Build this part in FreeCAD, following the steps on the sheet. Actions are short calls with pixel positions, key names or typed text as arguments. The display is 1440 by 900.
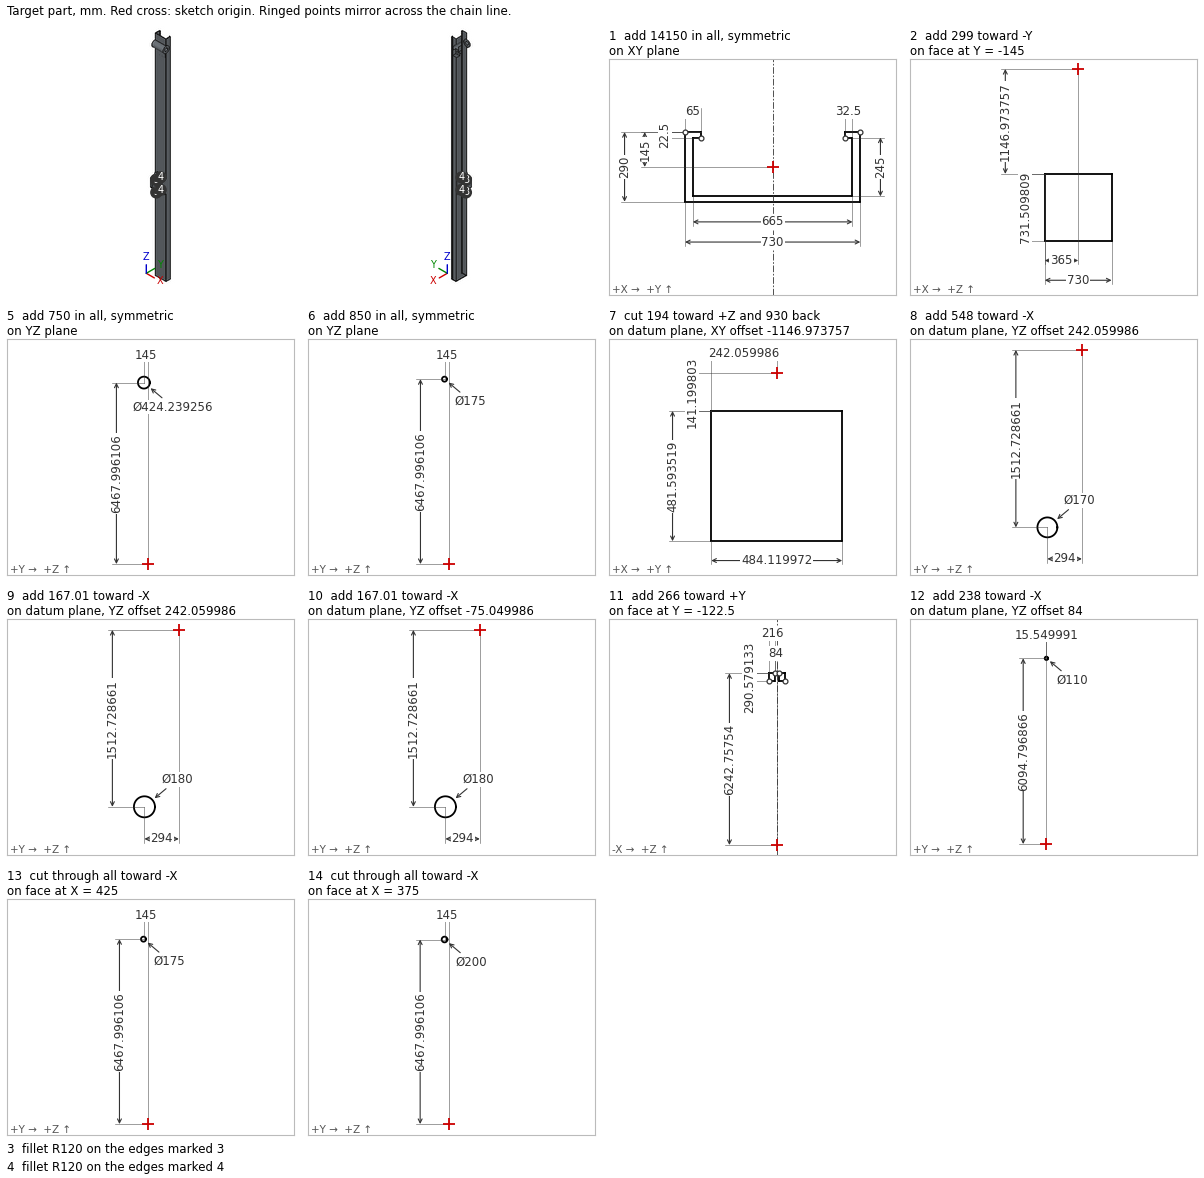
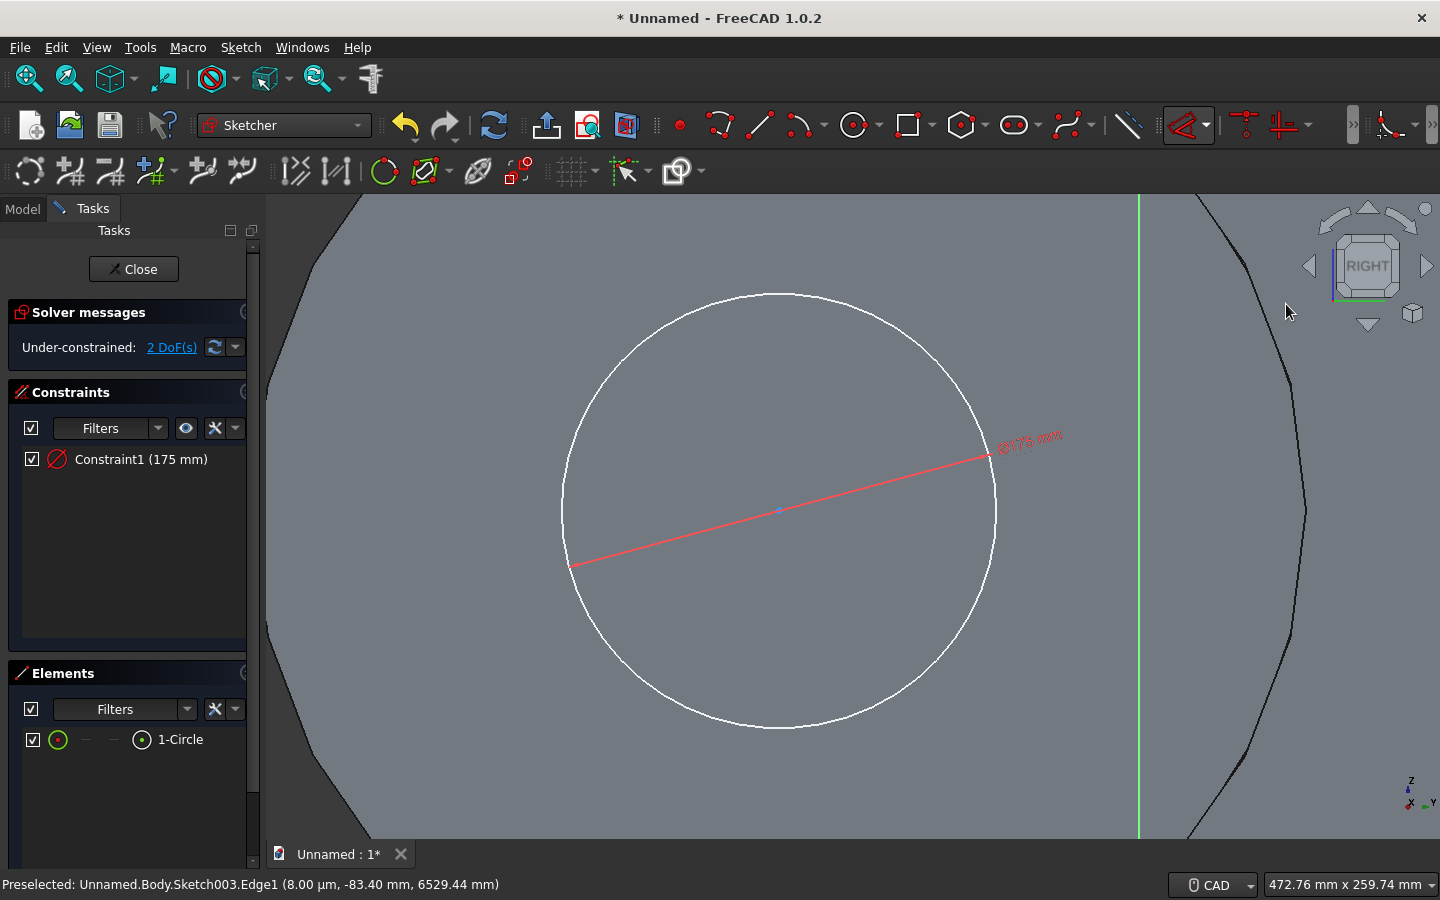
click(779, 511)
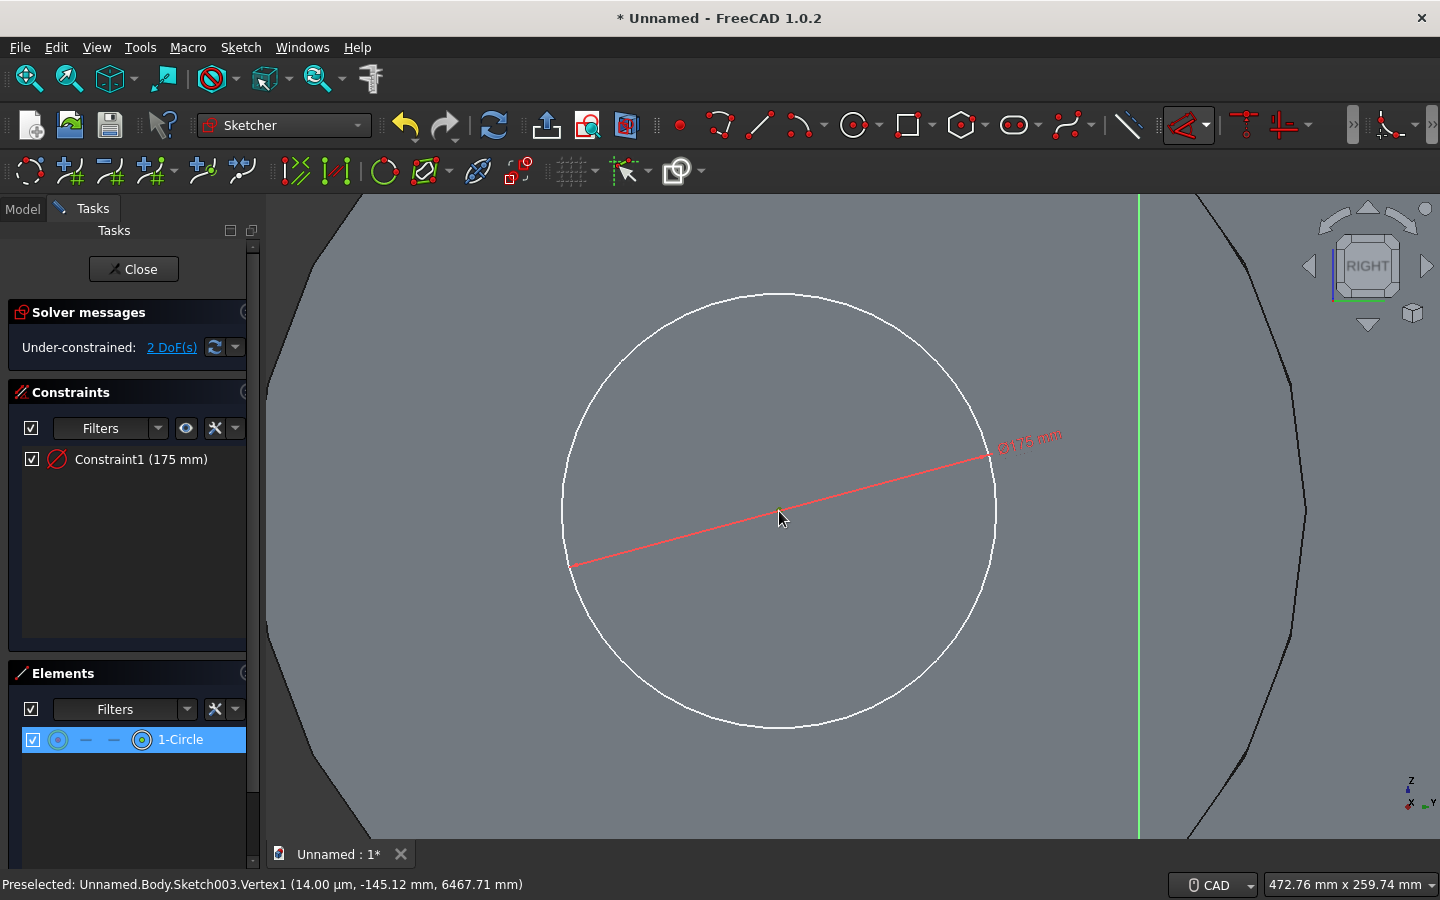
key(l)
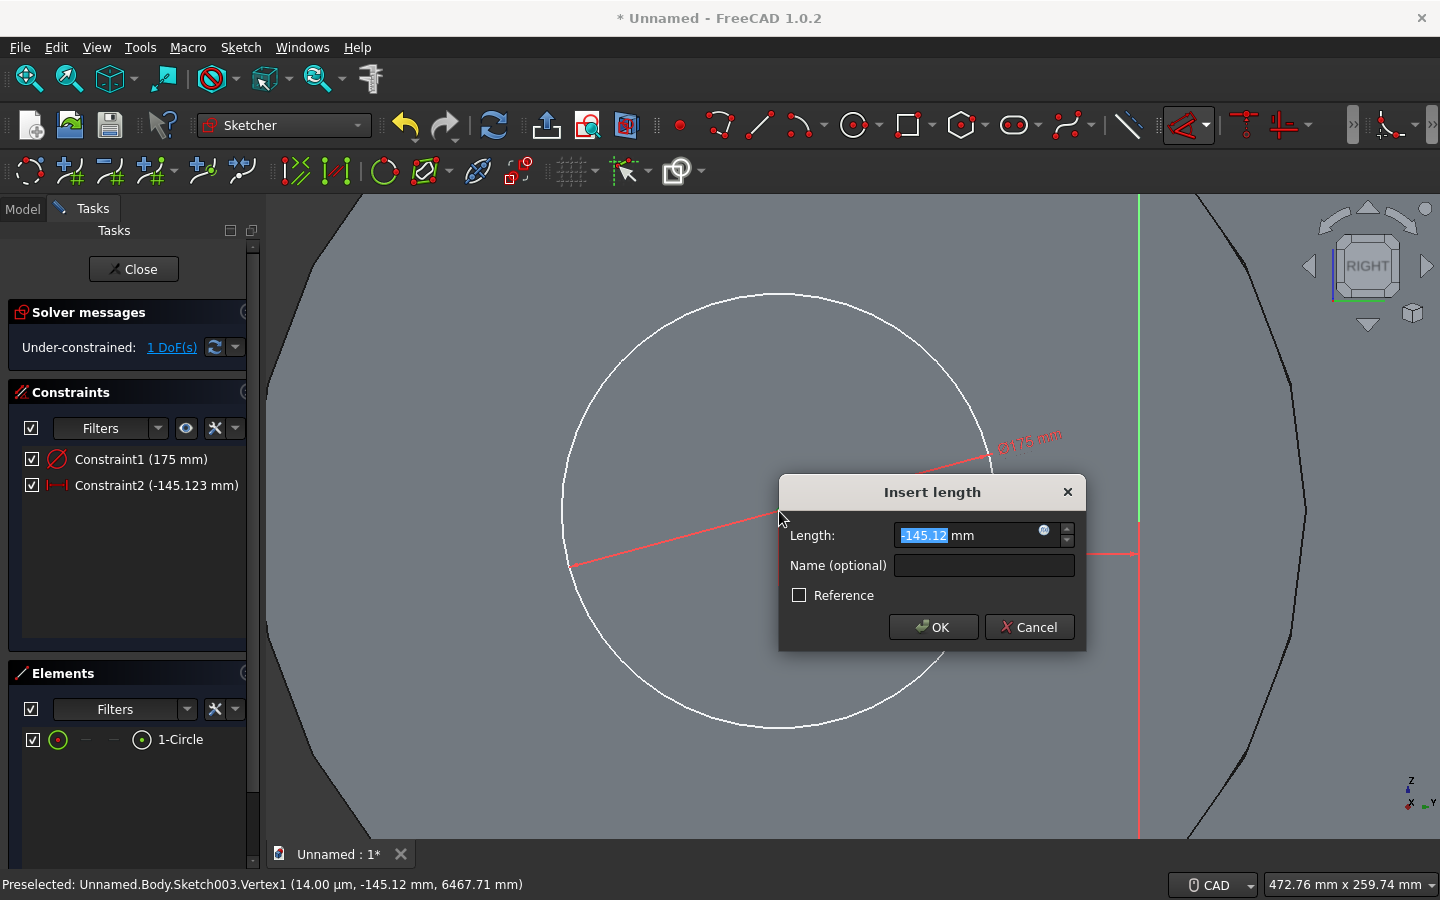
text(-145)
key(Return)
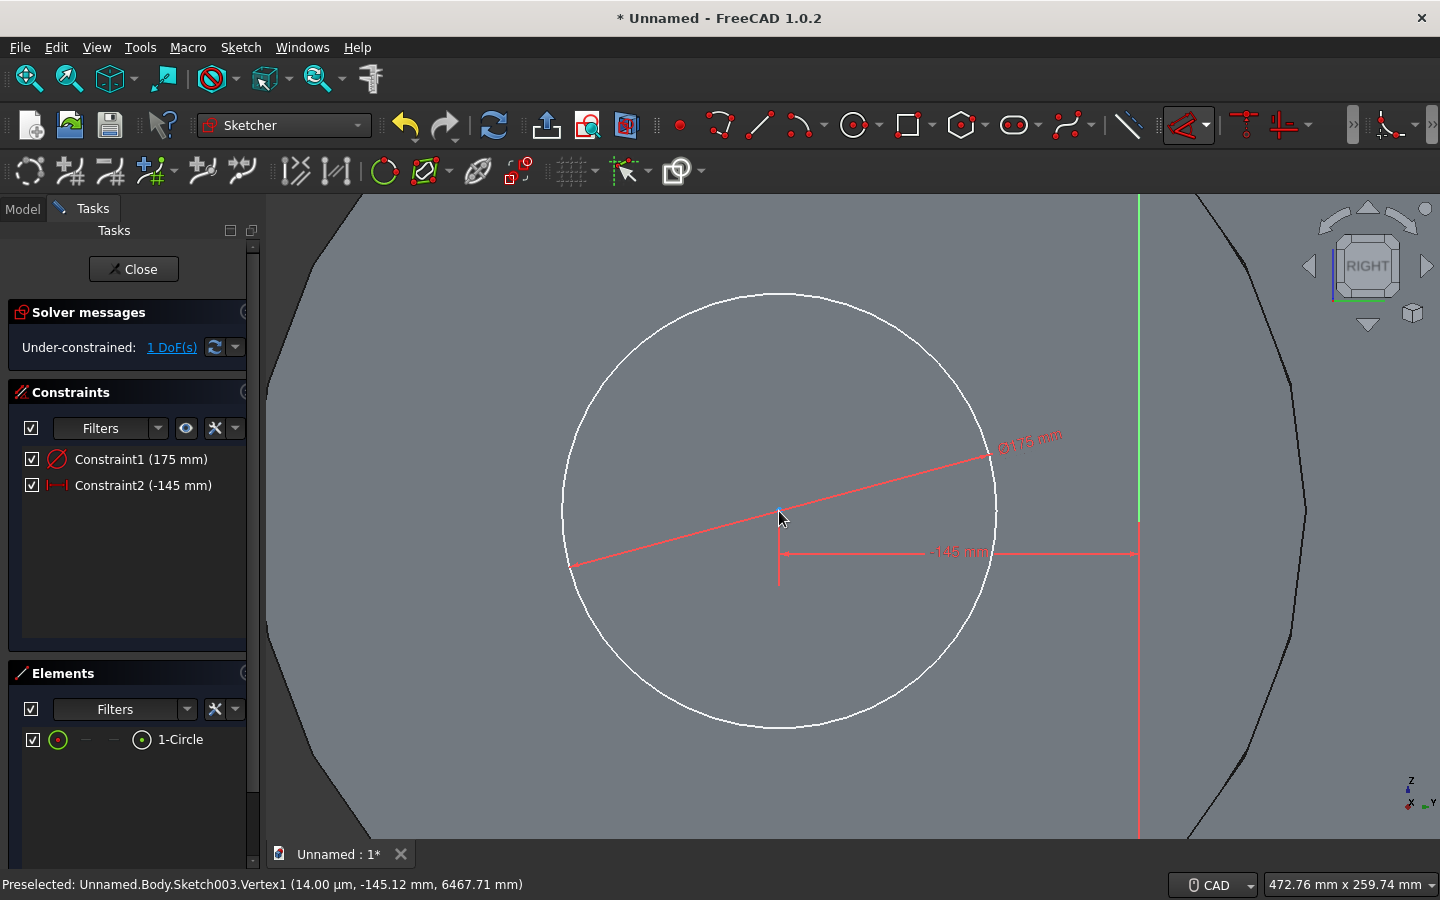
click(779, 511)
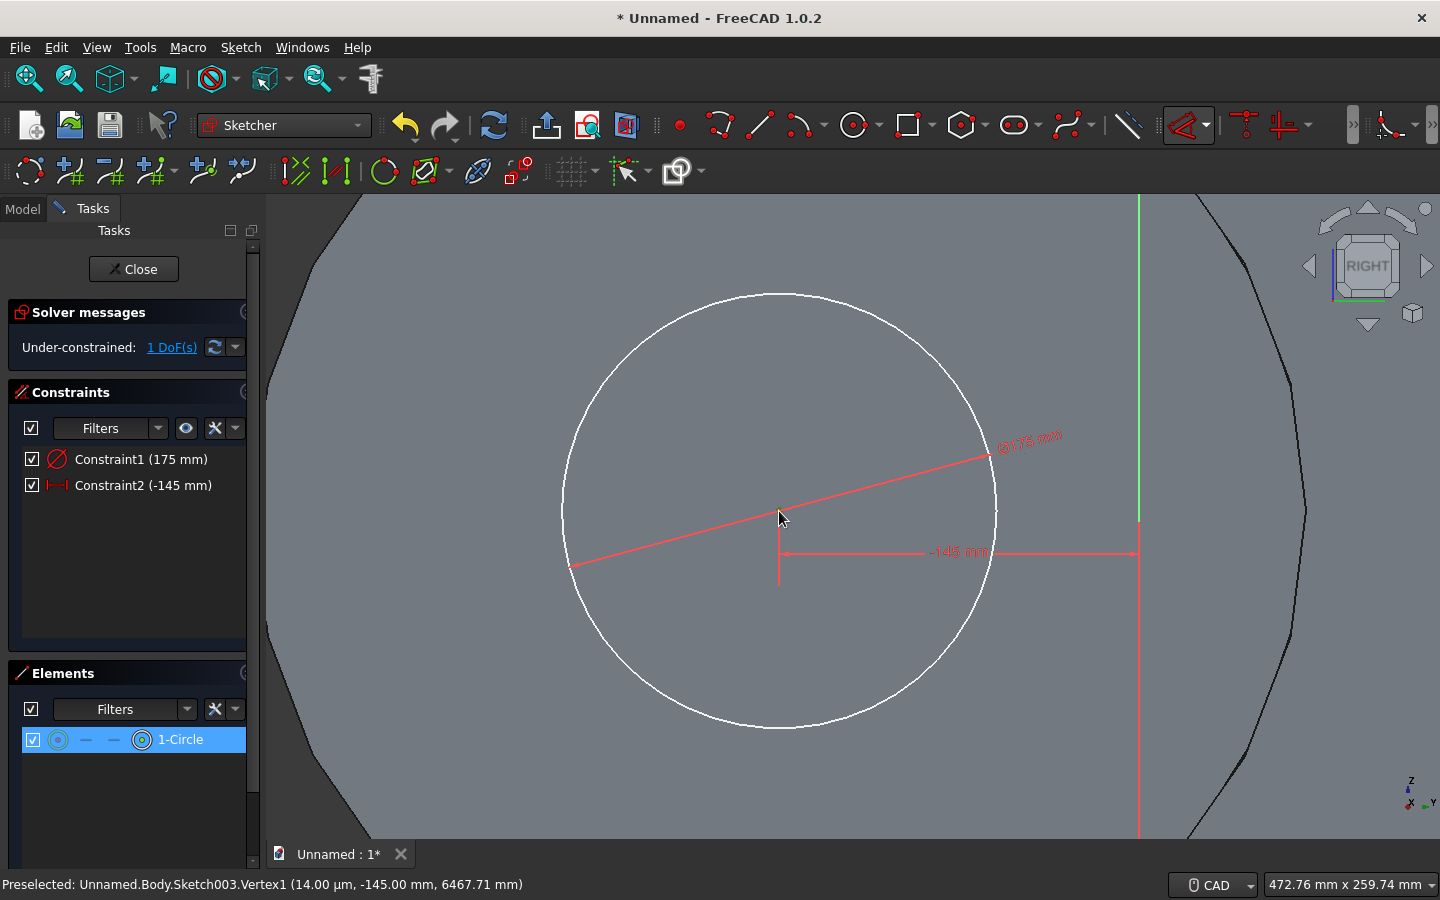
key(i)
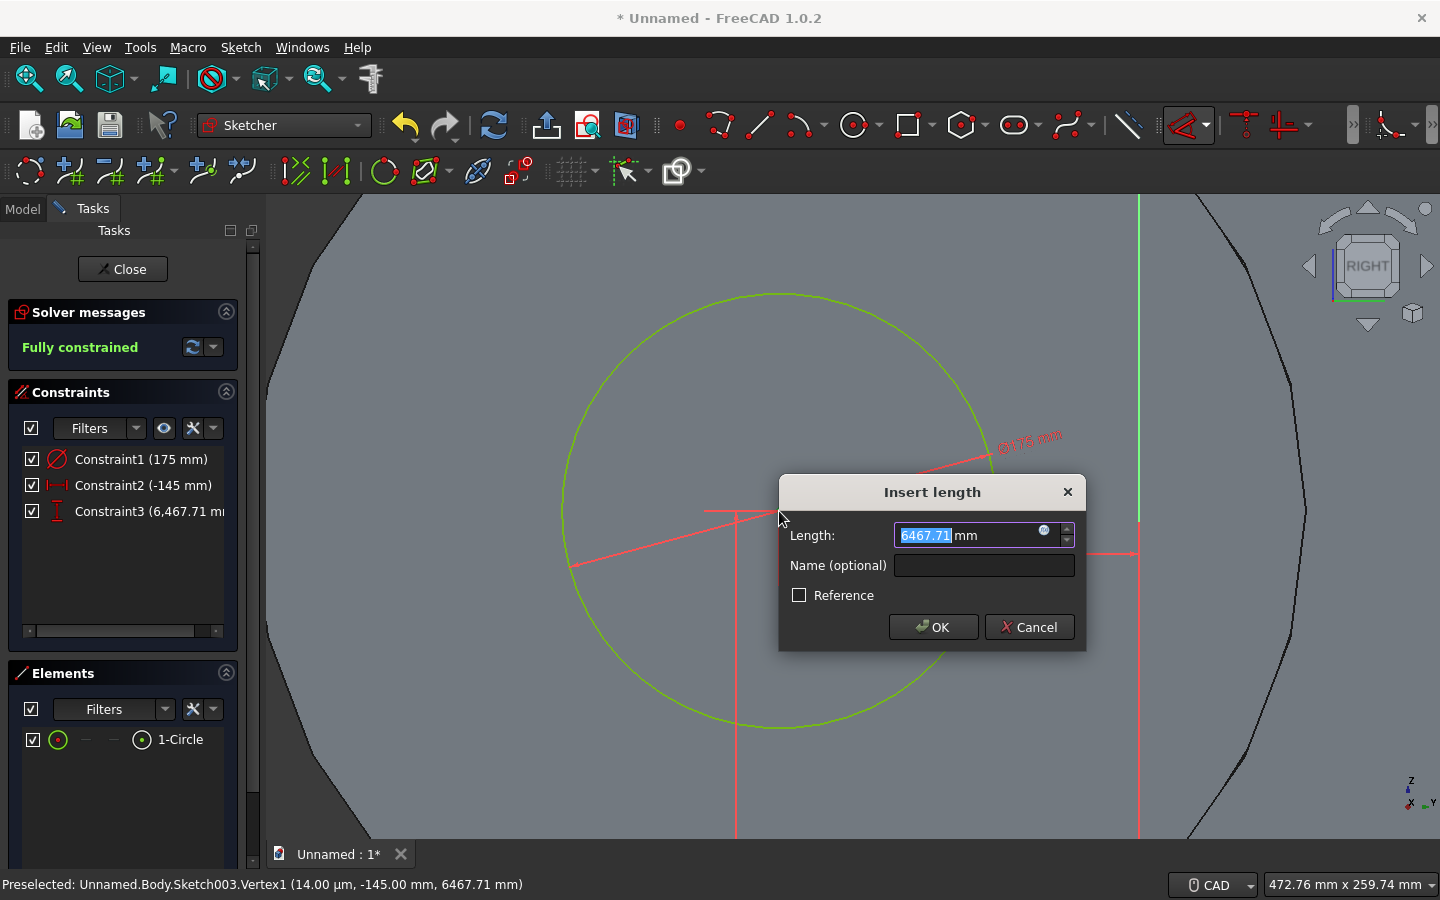
text(6467.996106)
key(Return)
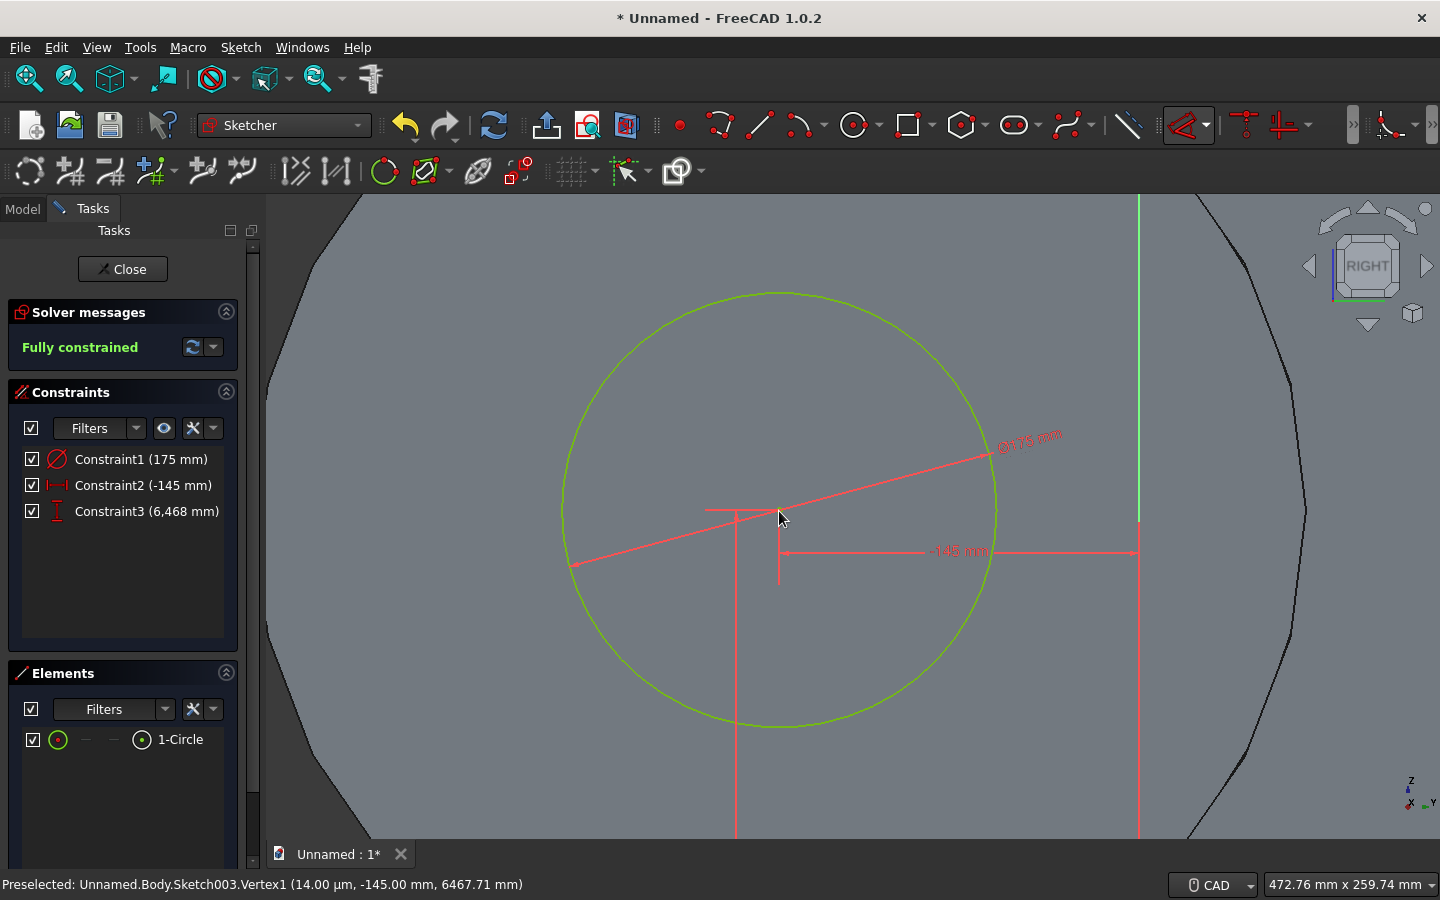
click(123, 269)